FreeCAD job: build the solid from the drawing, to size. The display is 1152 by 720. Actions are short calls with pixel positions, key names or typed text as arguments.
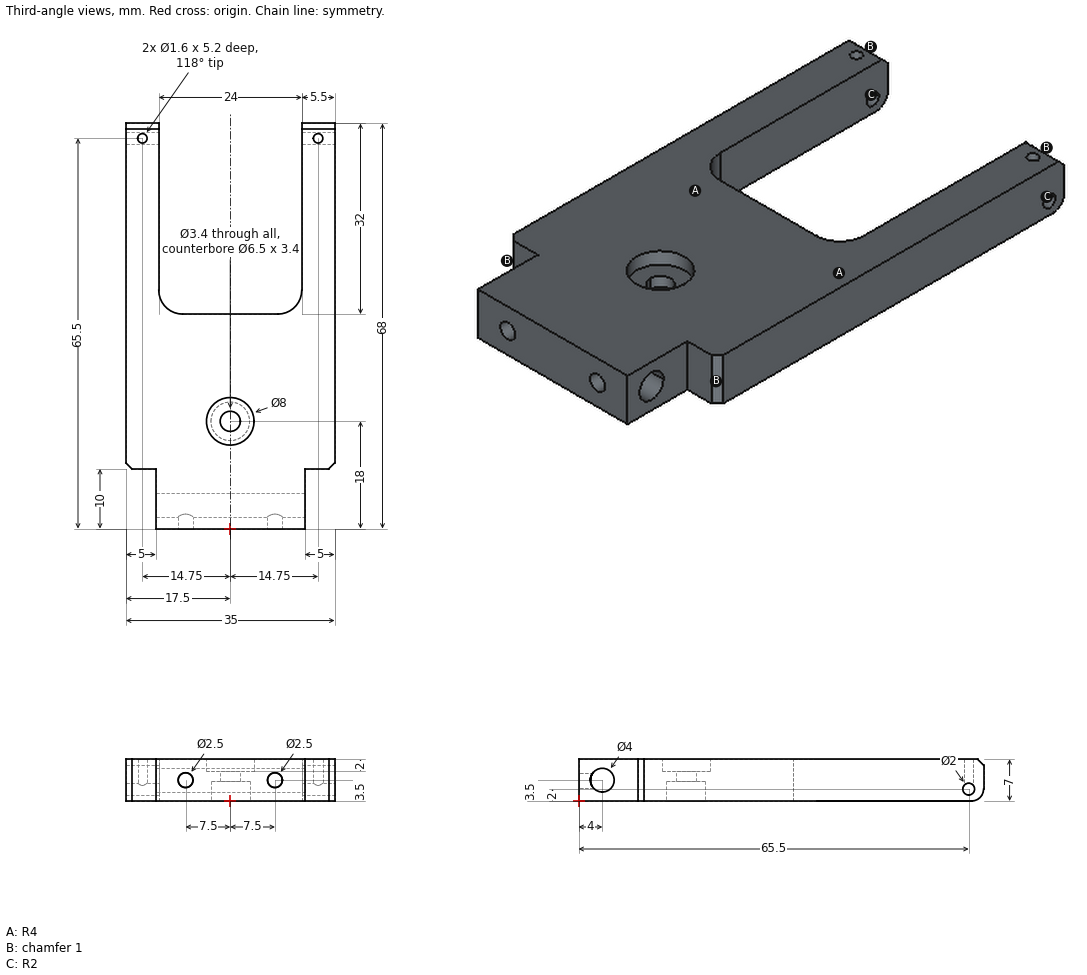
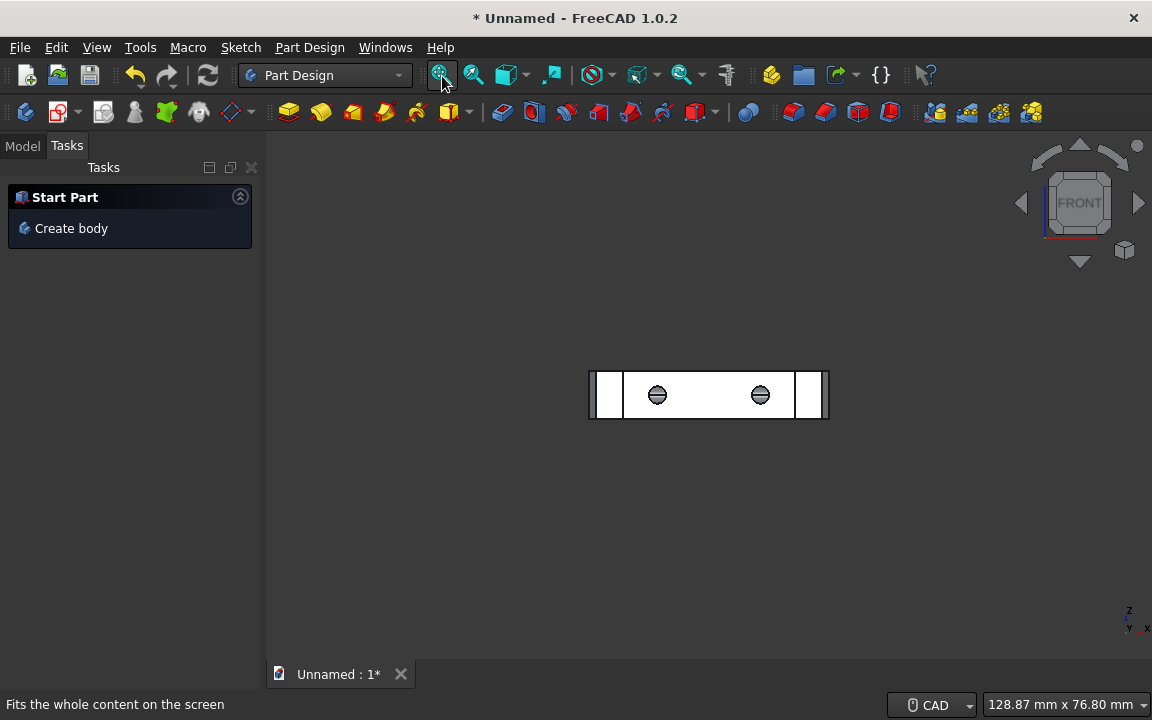
key(3)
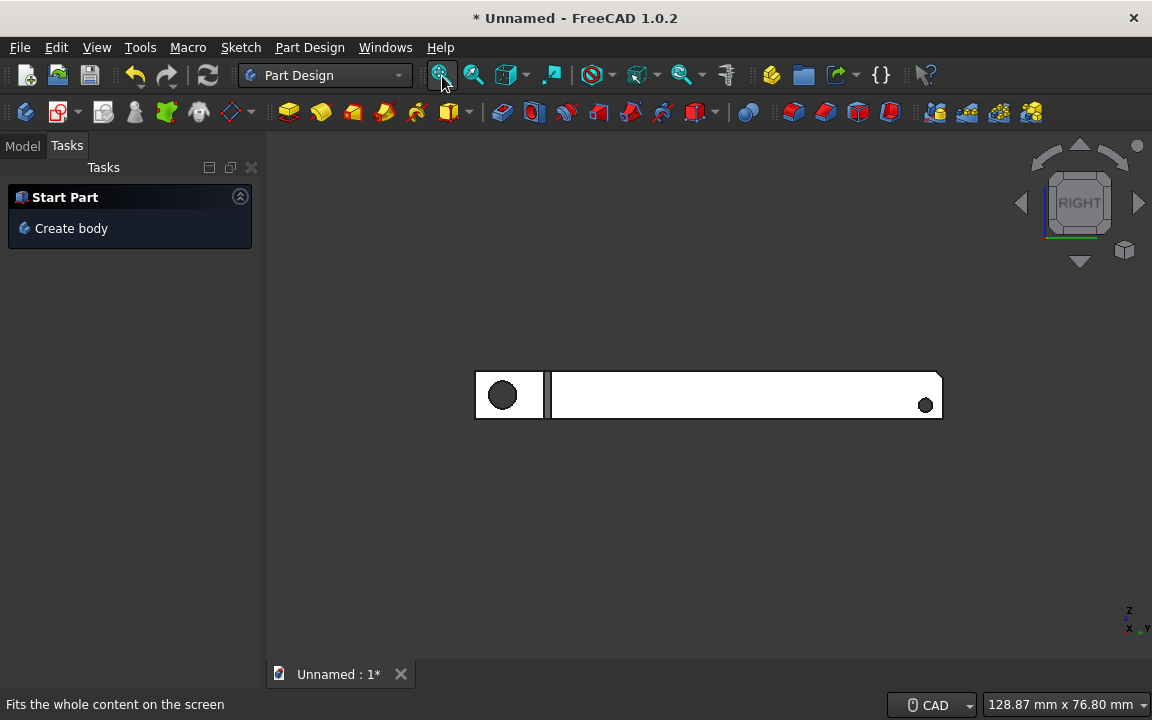
key(5)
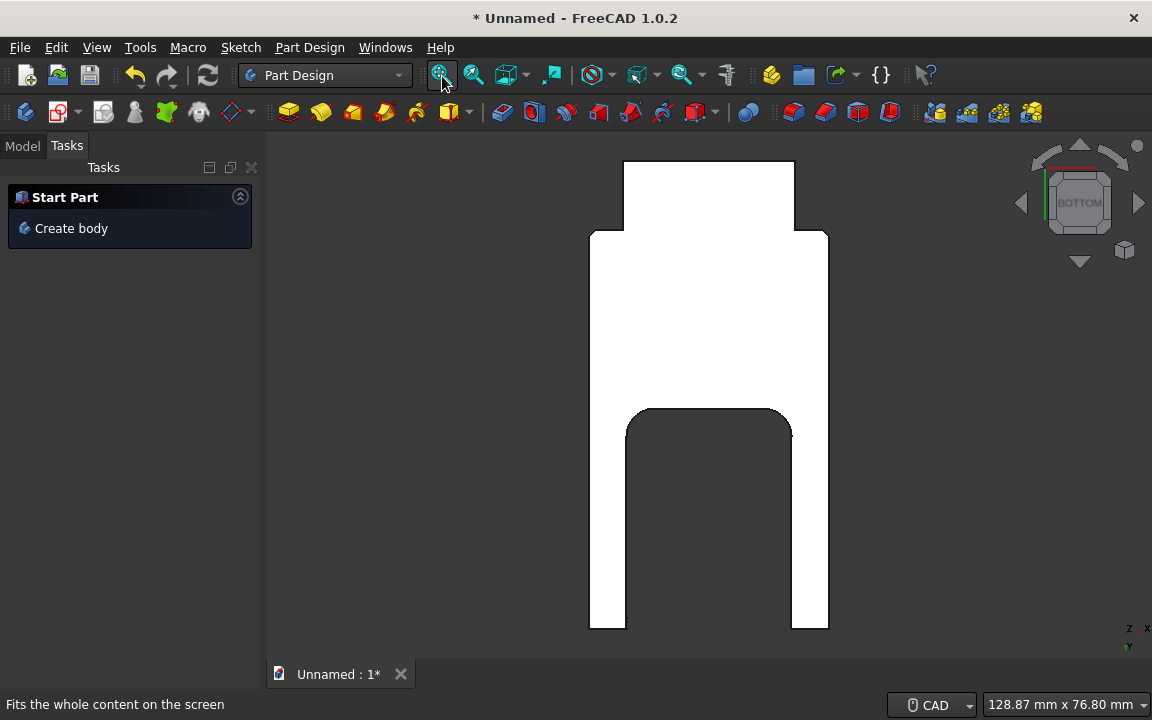
click(608, 628)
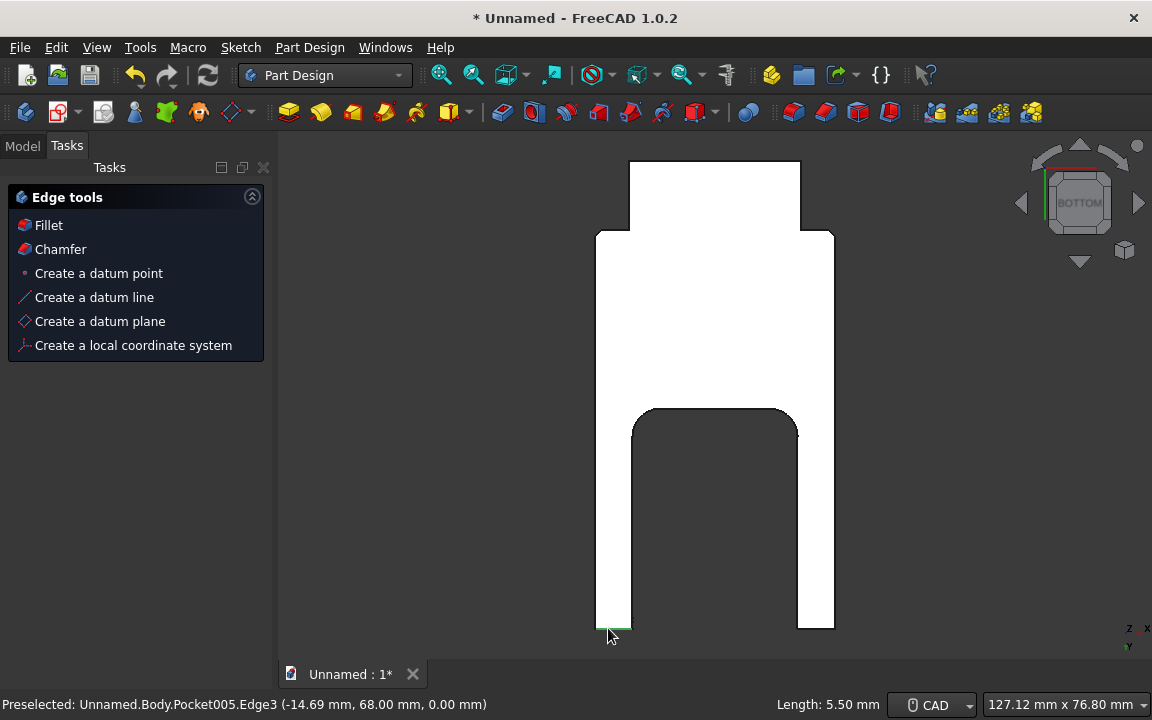
click(816, 628, ctrl)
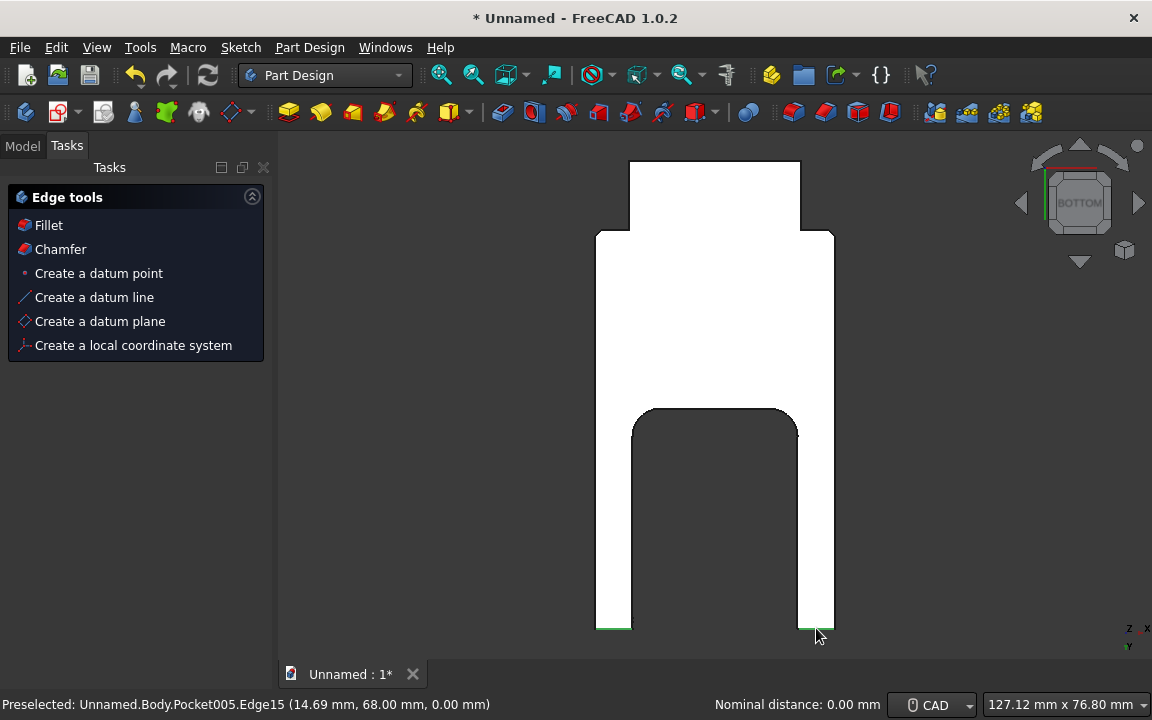
click(794, 112)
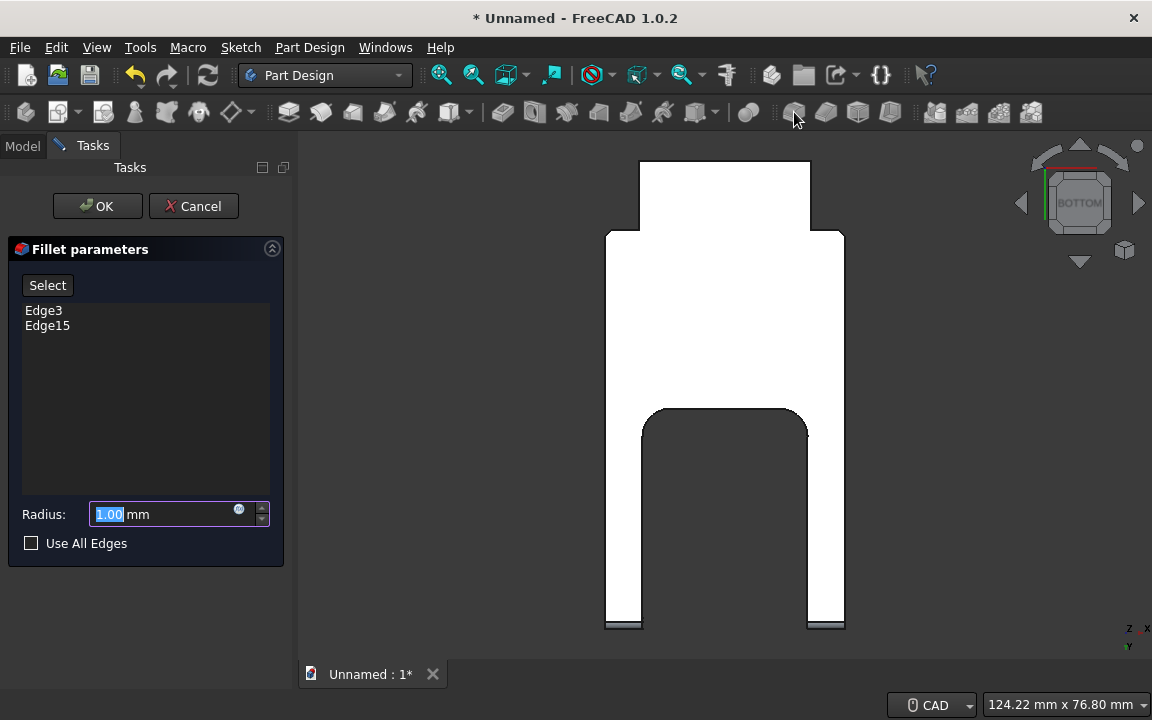
text(2)
key(Tab)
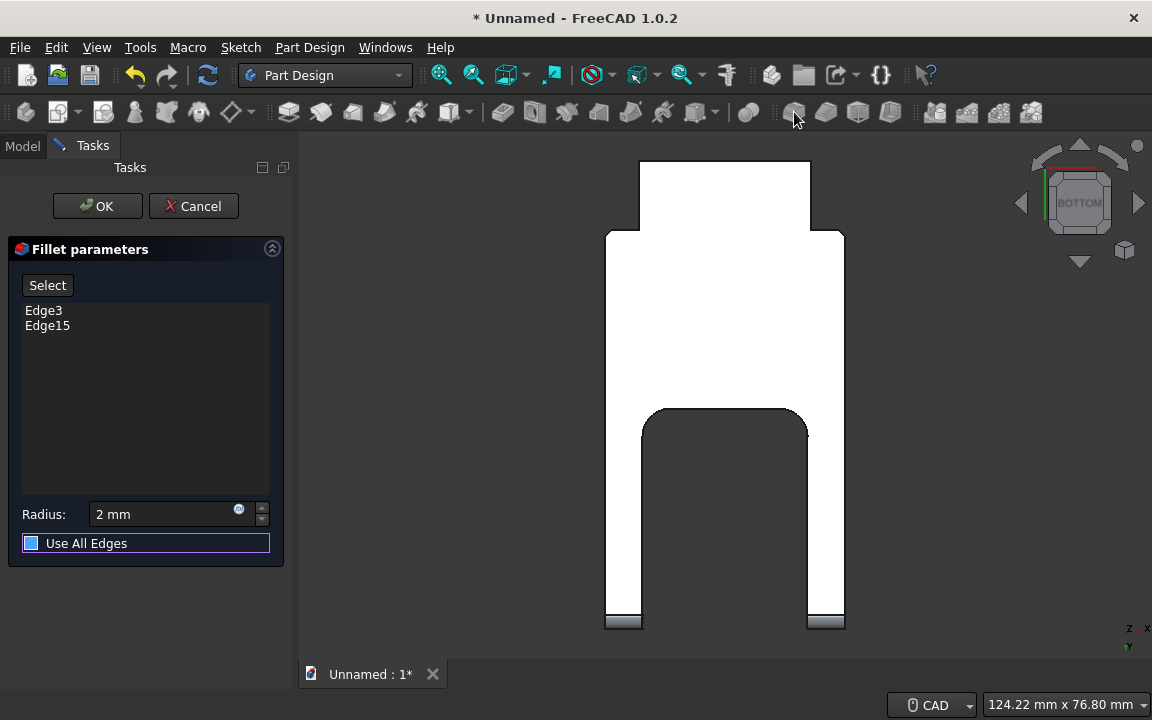
click(98, 206)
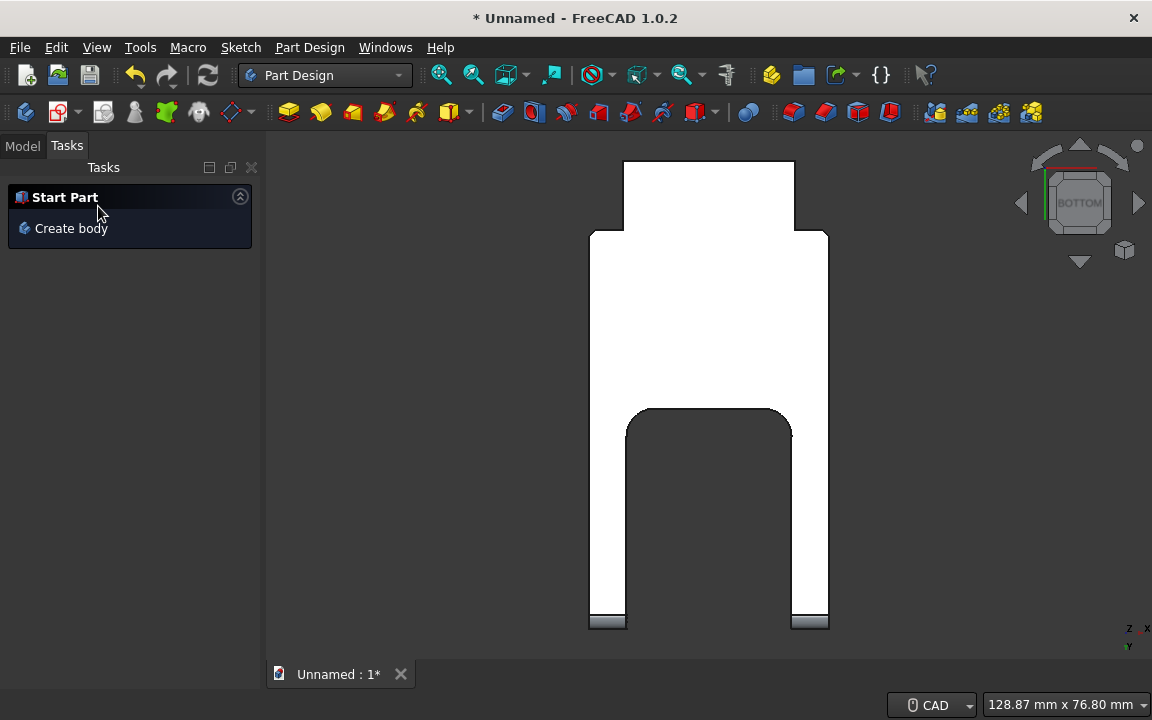
key(0)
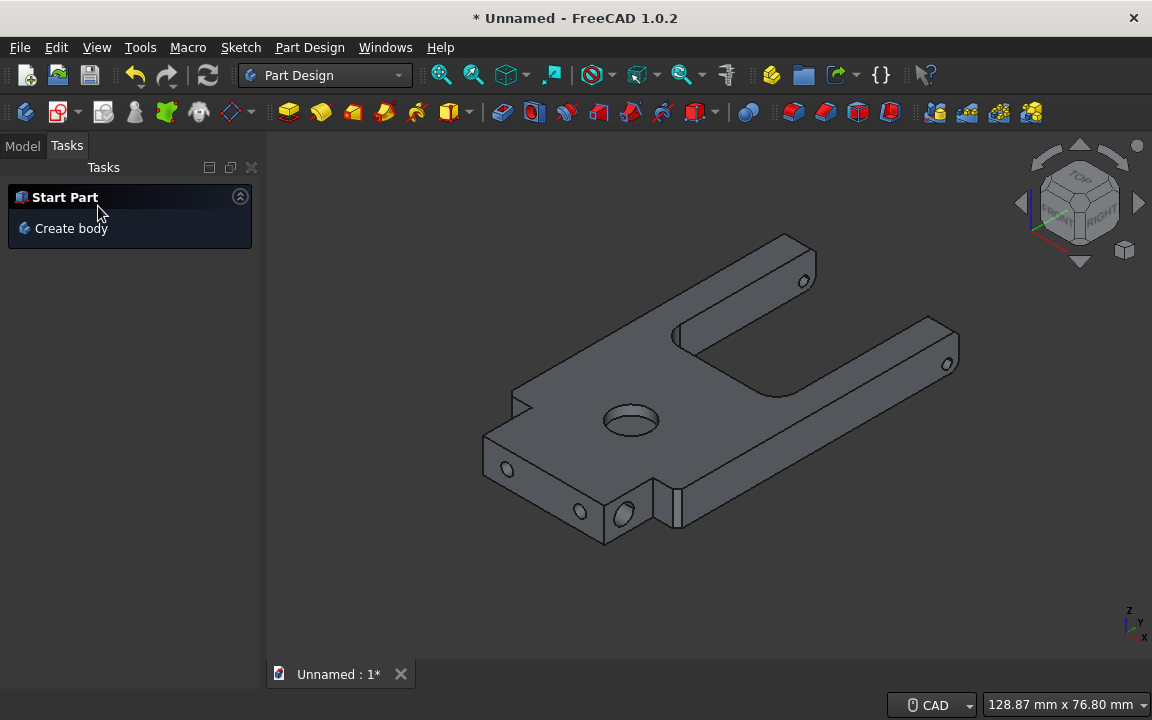
click(709, 431)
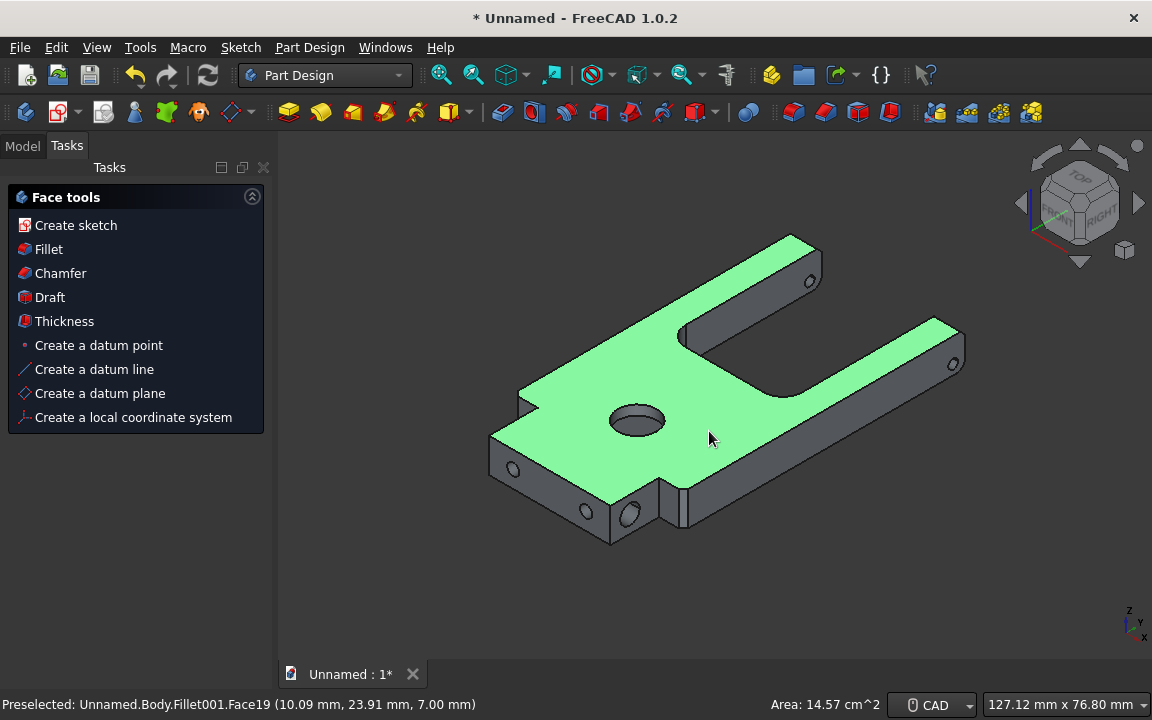
click(58, 112)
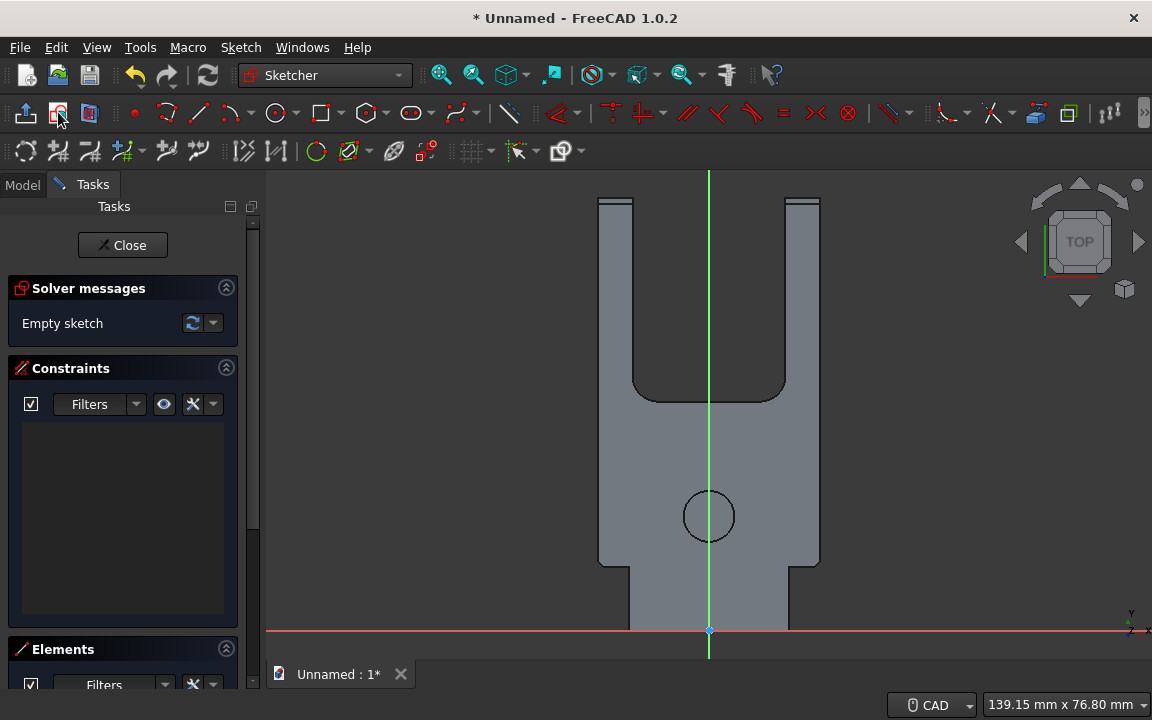
scroll(501, 403, down, 2)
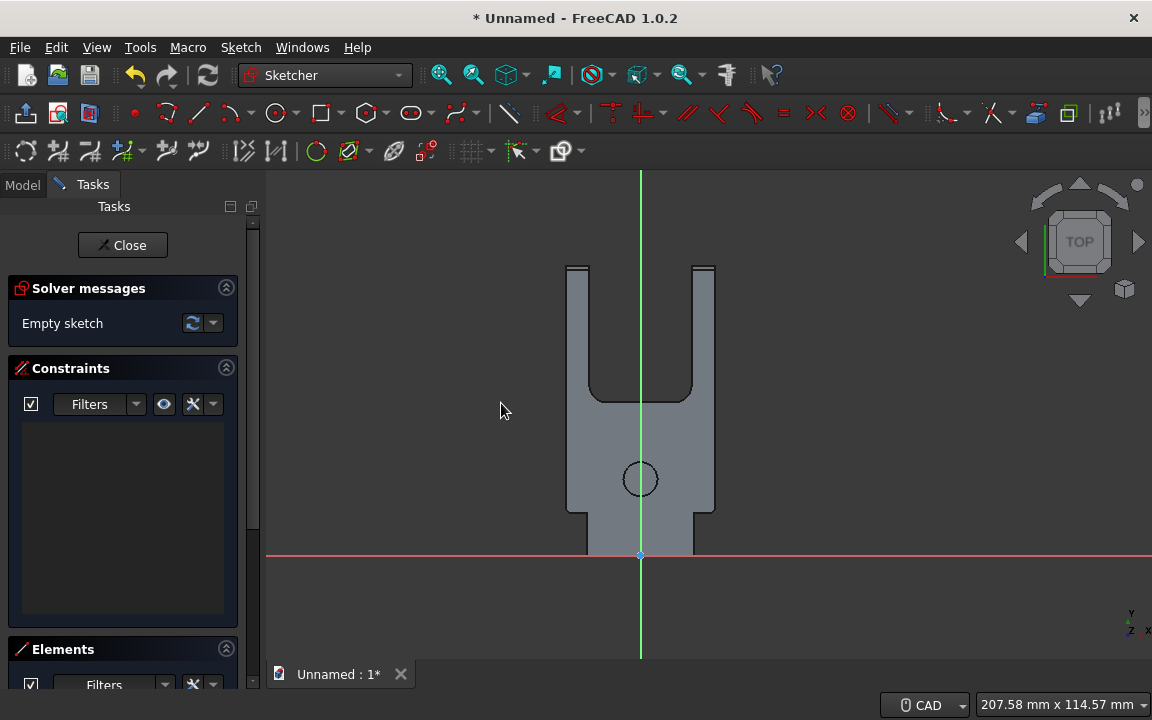
key(g)
key(c)